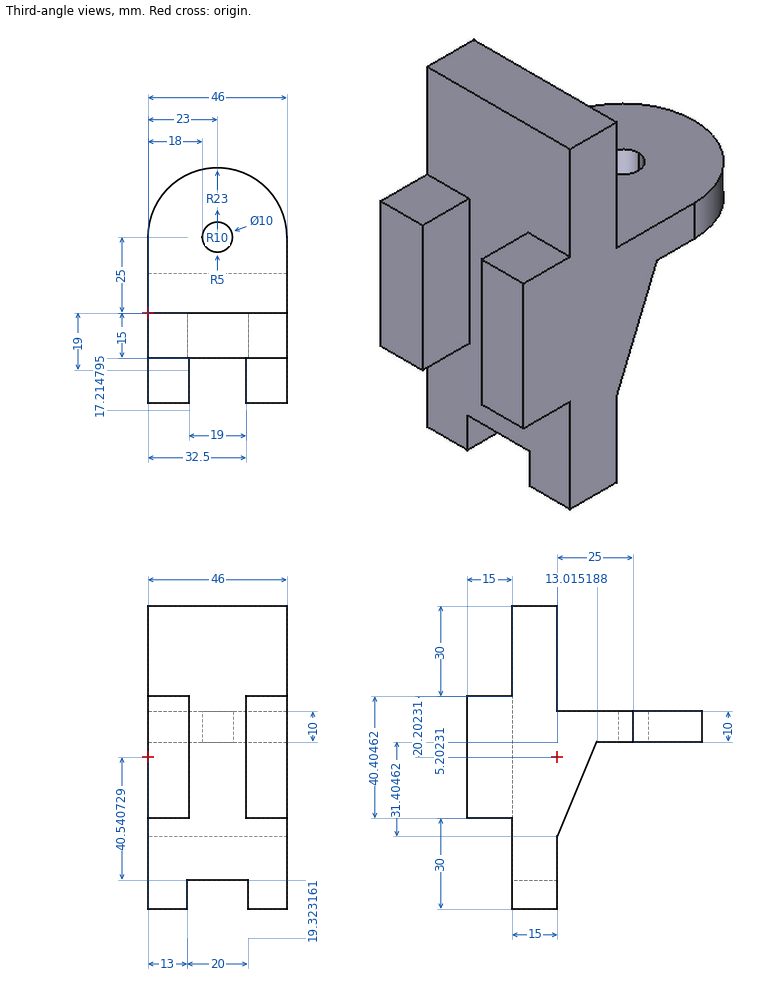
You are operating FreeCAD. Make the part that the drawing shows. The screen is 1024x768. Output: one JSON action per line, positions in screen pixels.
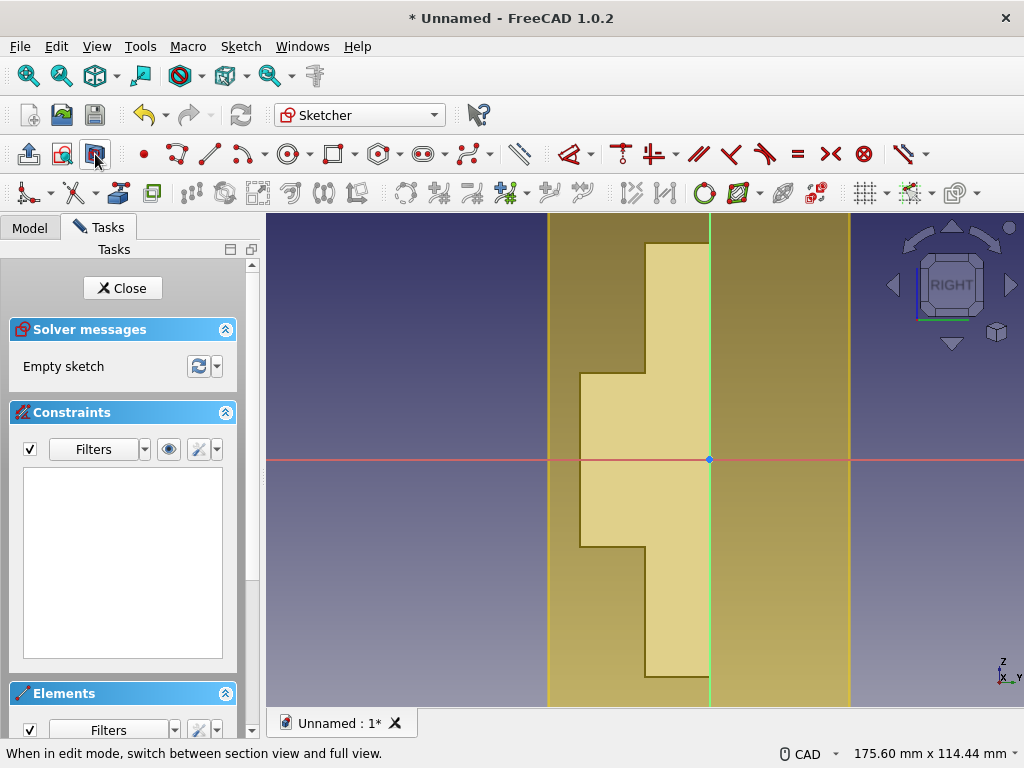
{"action": "scroll", "coordinate": [825, 416], "scroll_direction": "up", "scroll_amount": 7}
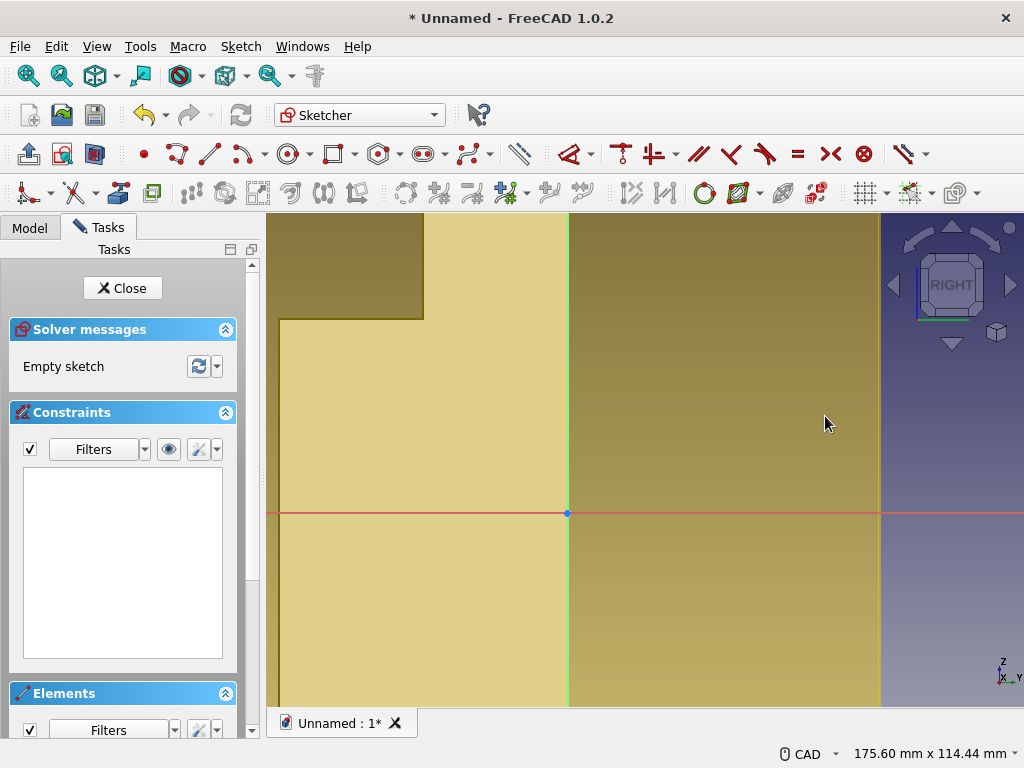
{"action": "key", "text": "g r"}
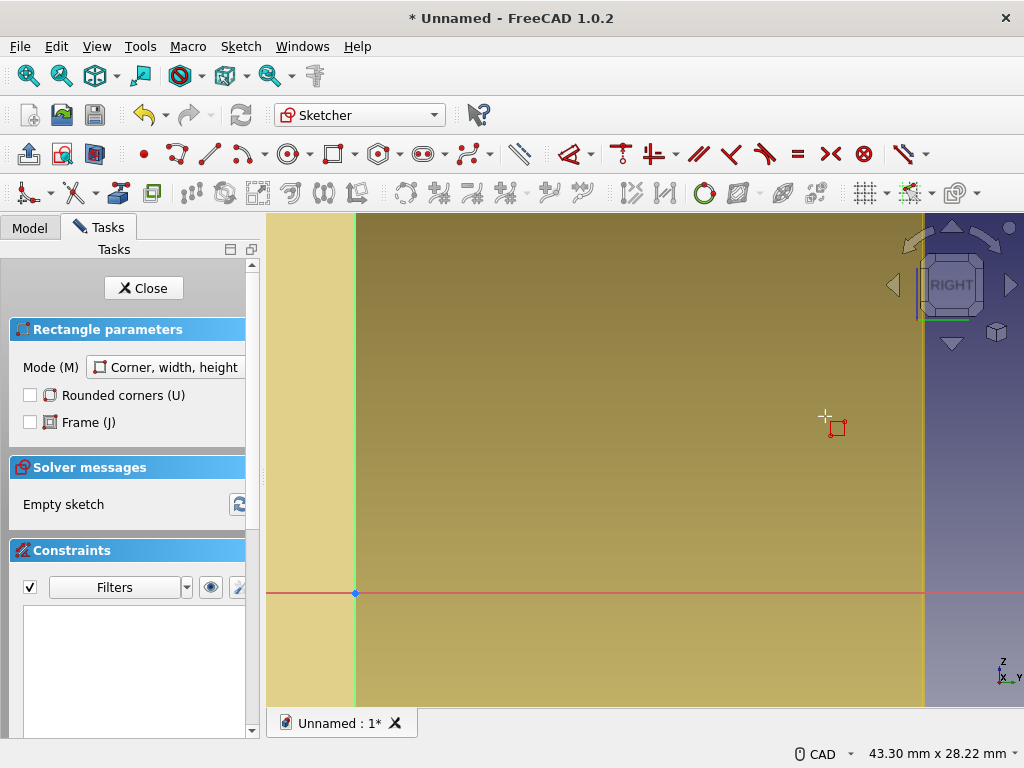
{"action": "left_click", "coordinate": [355, 327]}
{"action": "mouse_move", "coordinate": [793, 502]}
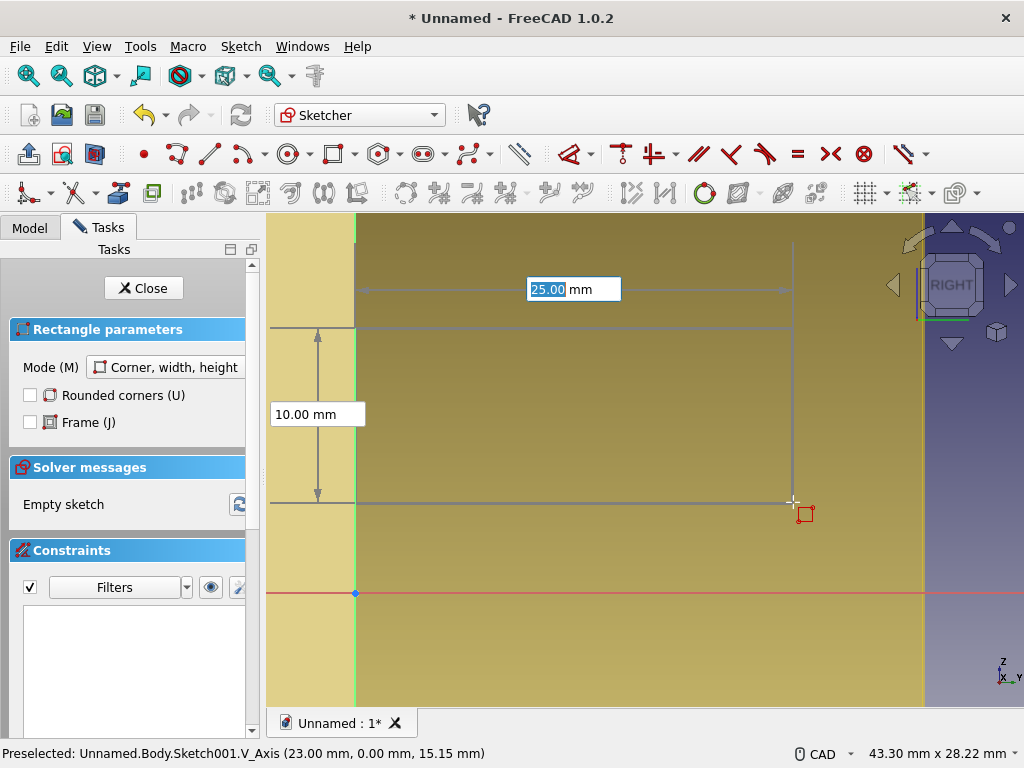
{"action": "type", "text": "25"}
{"action": "key", "text": "Tab"}
{"action": "type", "text": "10"}
{"action": "key", "text": "Return"}
{"action": "key", "text": "Escape"}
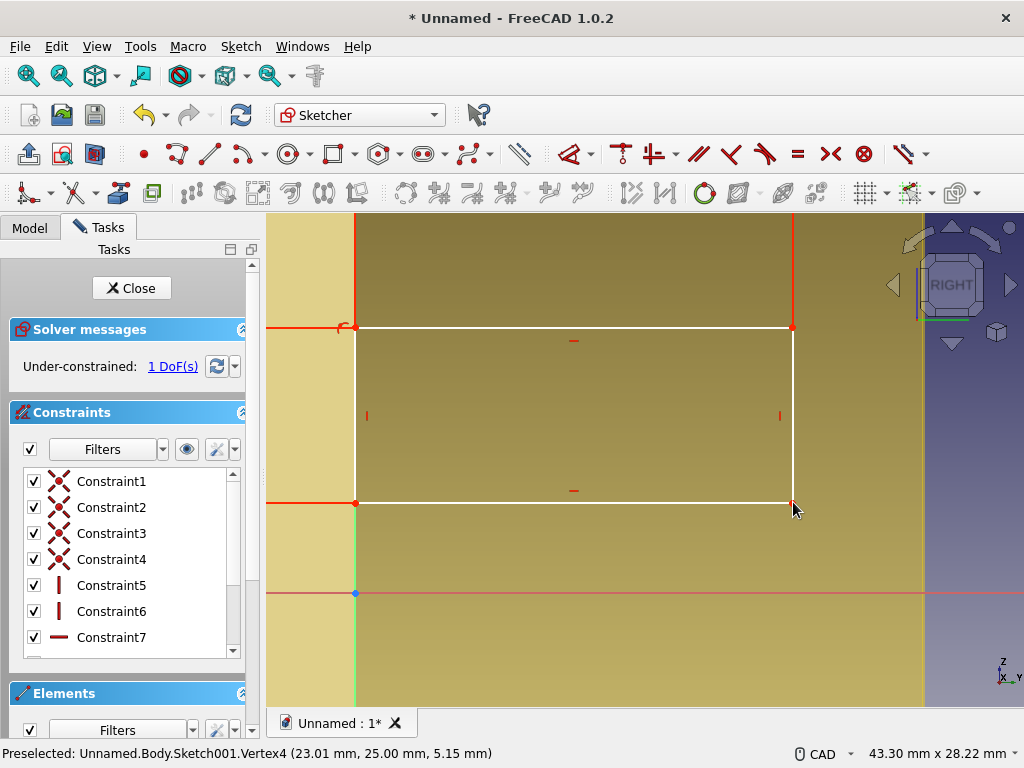
{"action": "key", "text": "d"}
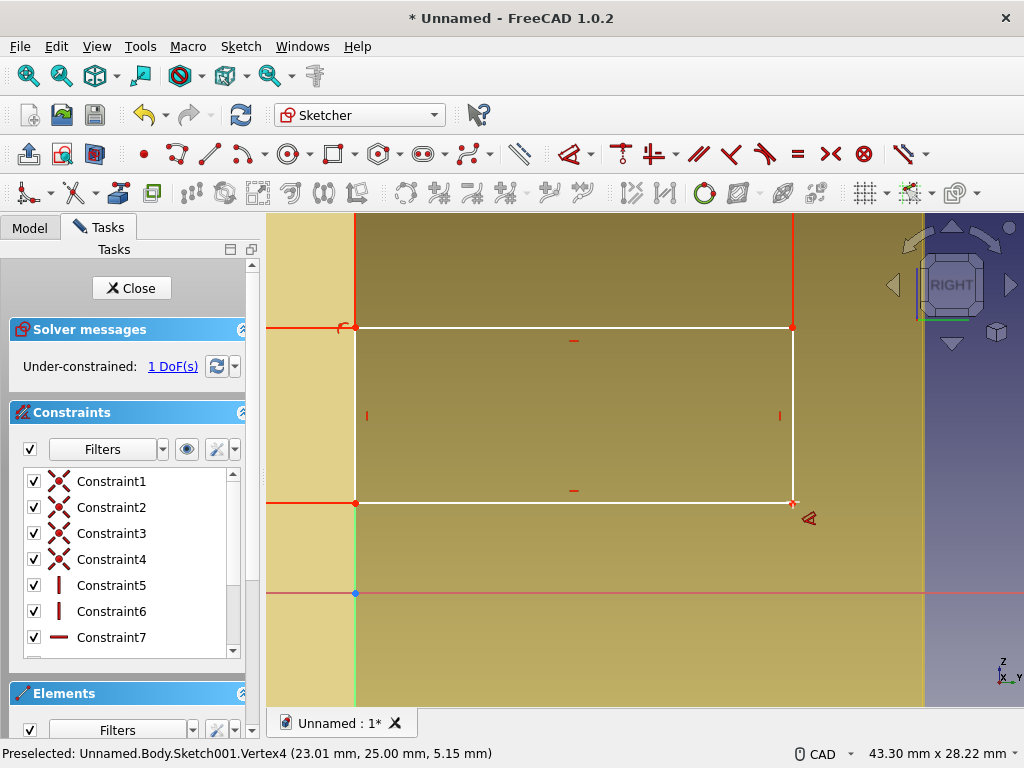
{"action": "left_click", "coordinate": [355, 503]}
{"action": "left_click", "coordinate": [321, 548]}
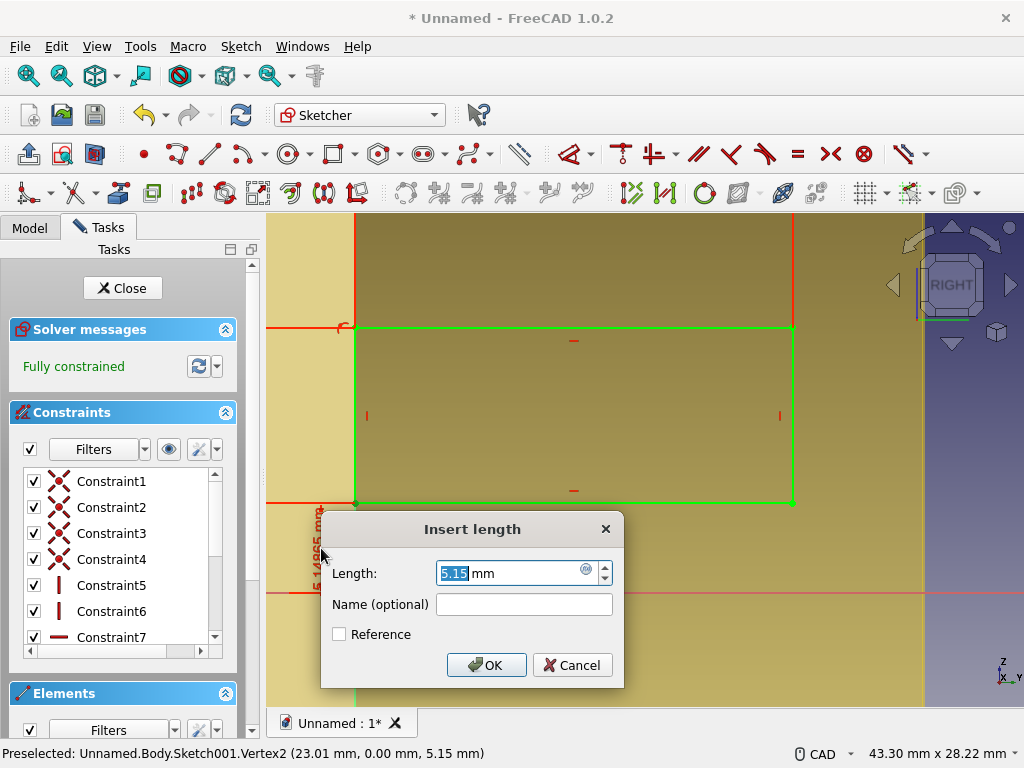
{"action": "type", "text": "5.20231"}
{"action": "key", "text": "Return"}
{"action": "key", "text": "Escape"}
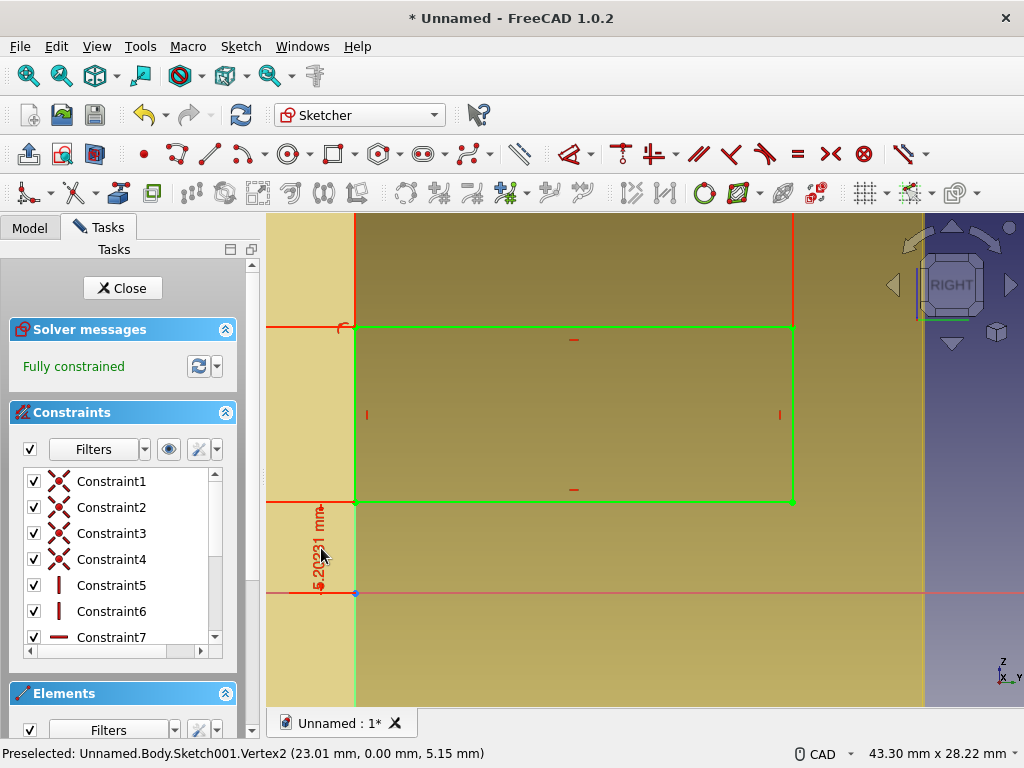
{"action": "left_click", "coordinate": [123, 288]}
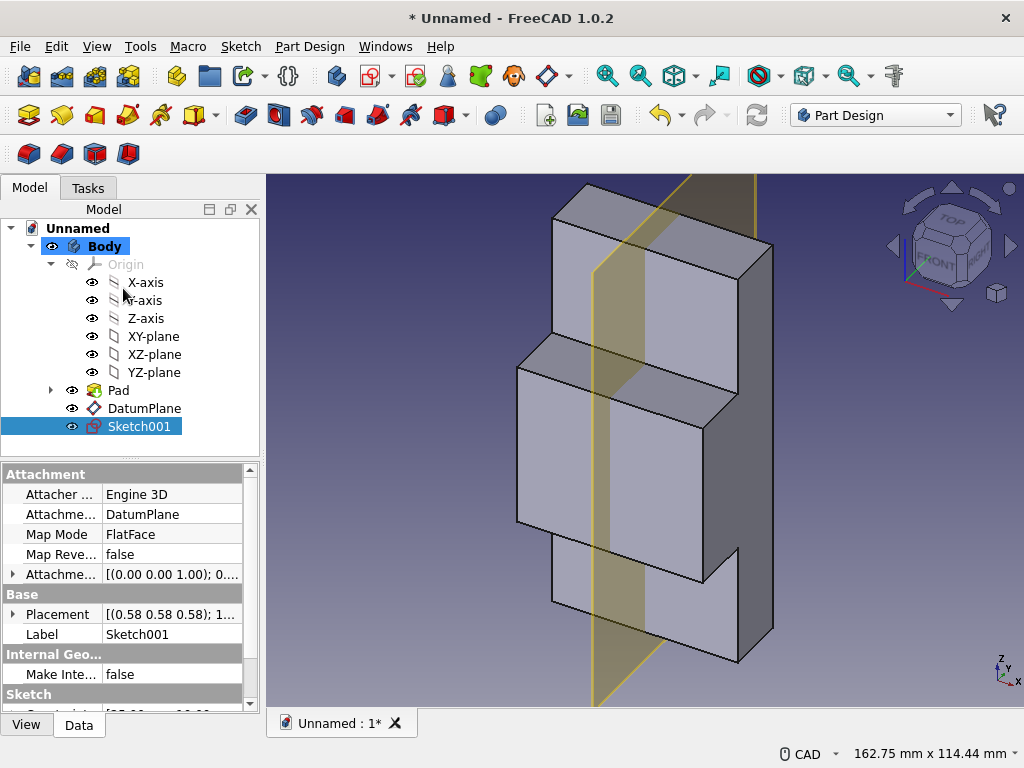
{"action": "left_click", "coordinate": [29, 116]}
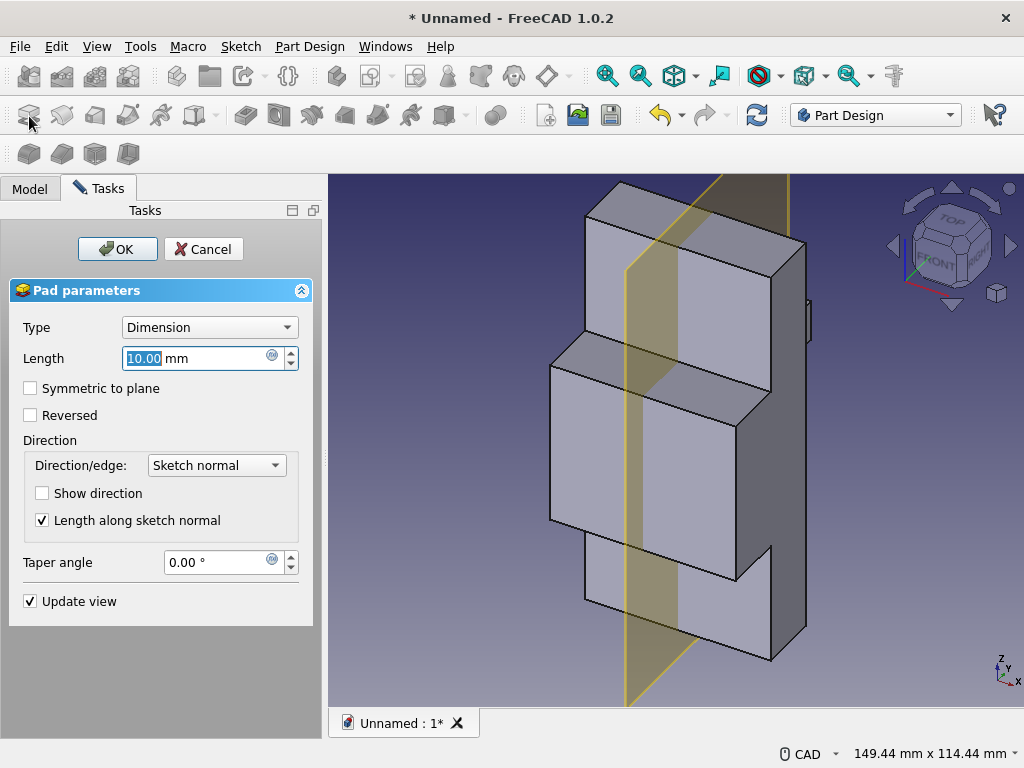
{"action": "type", "text": "46"}
{"action": "key", "text": "Tab"}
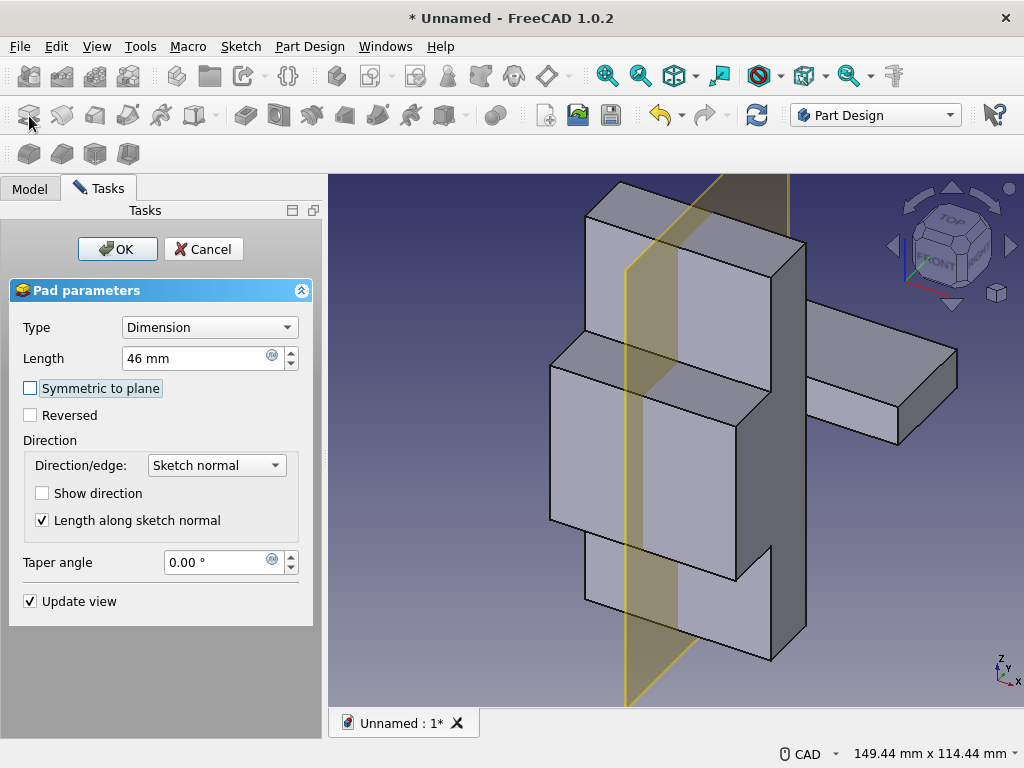
{"action": "left_click", "coordinate": [31, 388]}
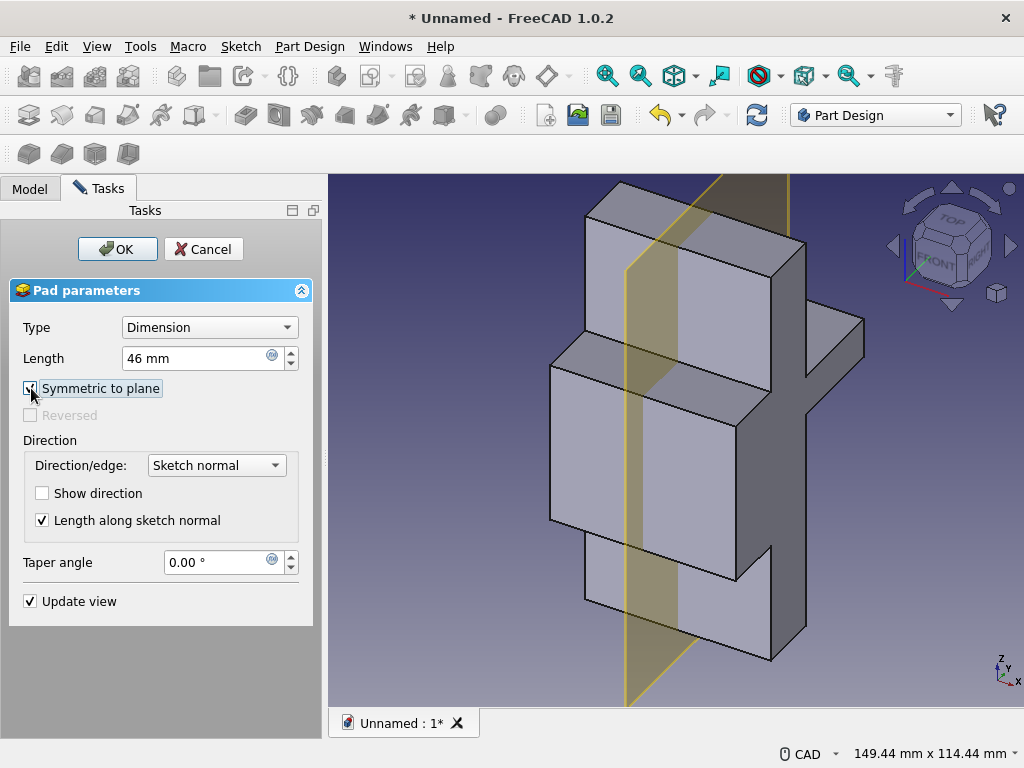
{"action": "left_click", "coordinate": [118, 249]}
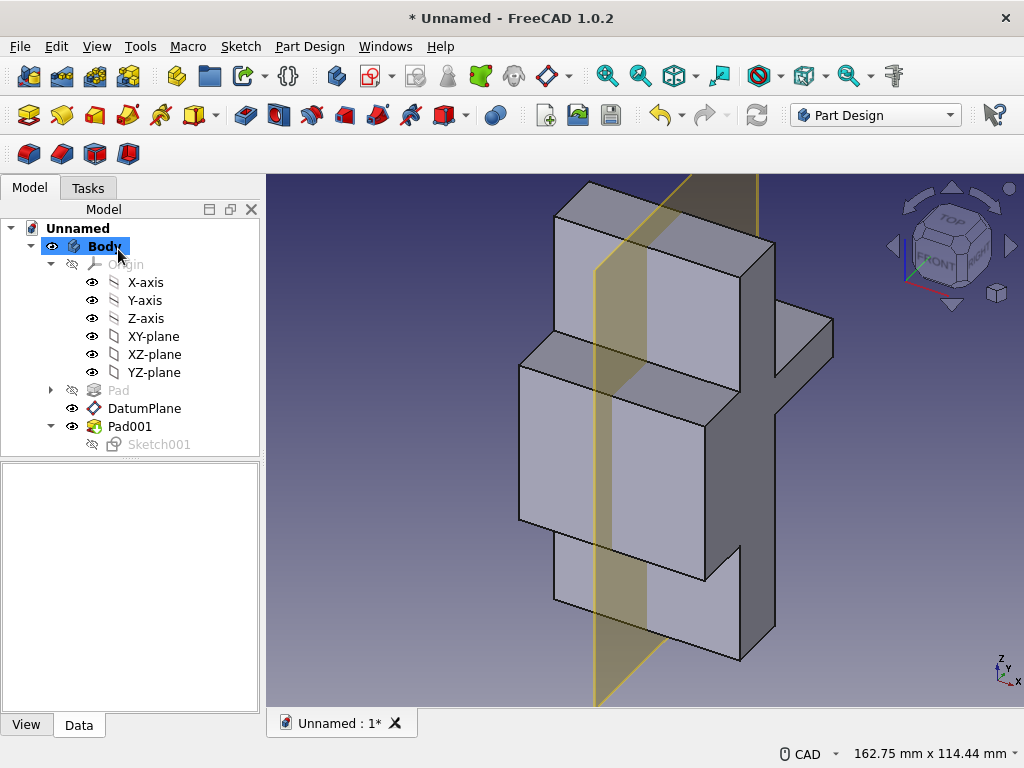
{"action": "left_click", "coordinate": [117, 408]}
{"action": "key", "text": "space"}